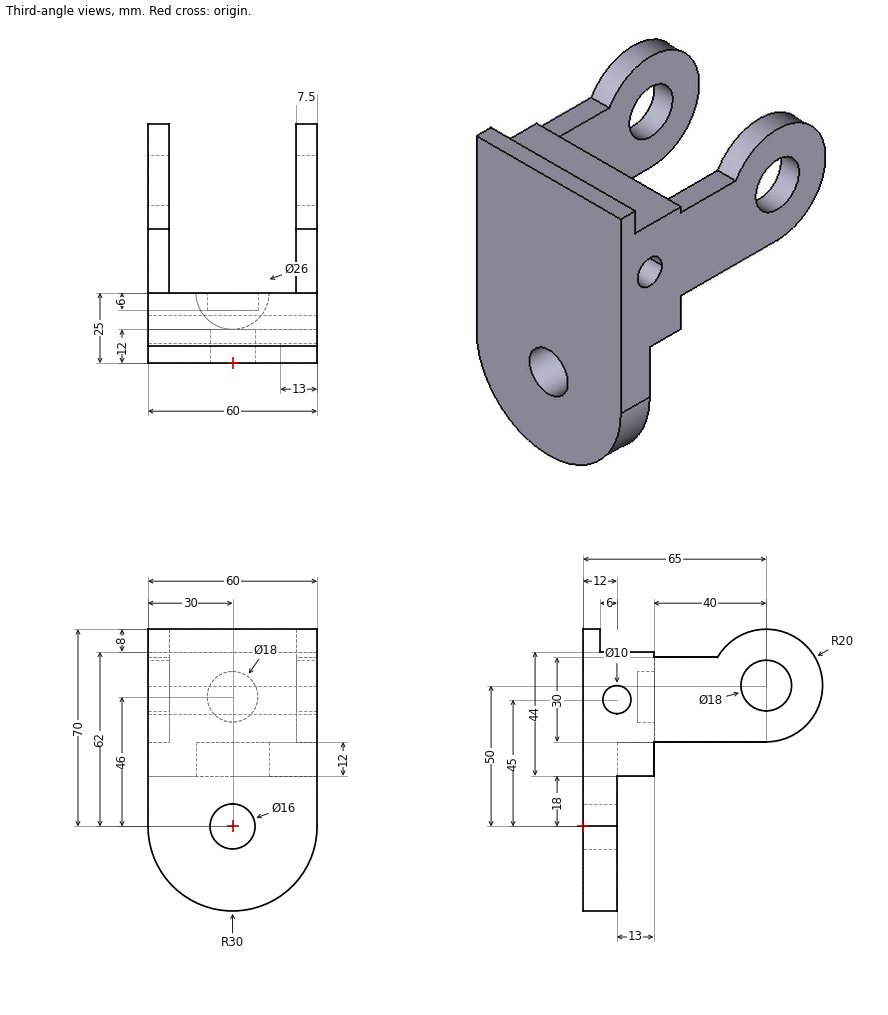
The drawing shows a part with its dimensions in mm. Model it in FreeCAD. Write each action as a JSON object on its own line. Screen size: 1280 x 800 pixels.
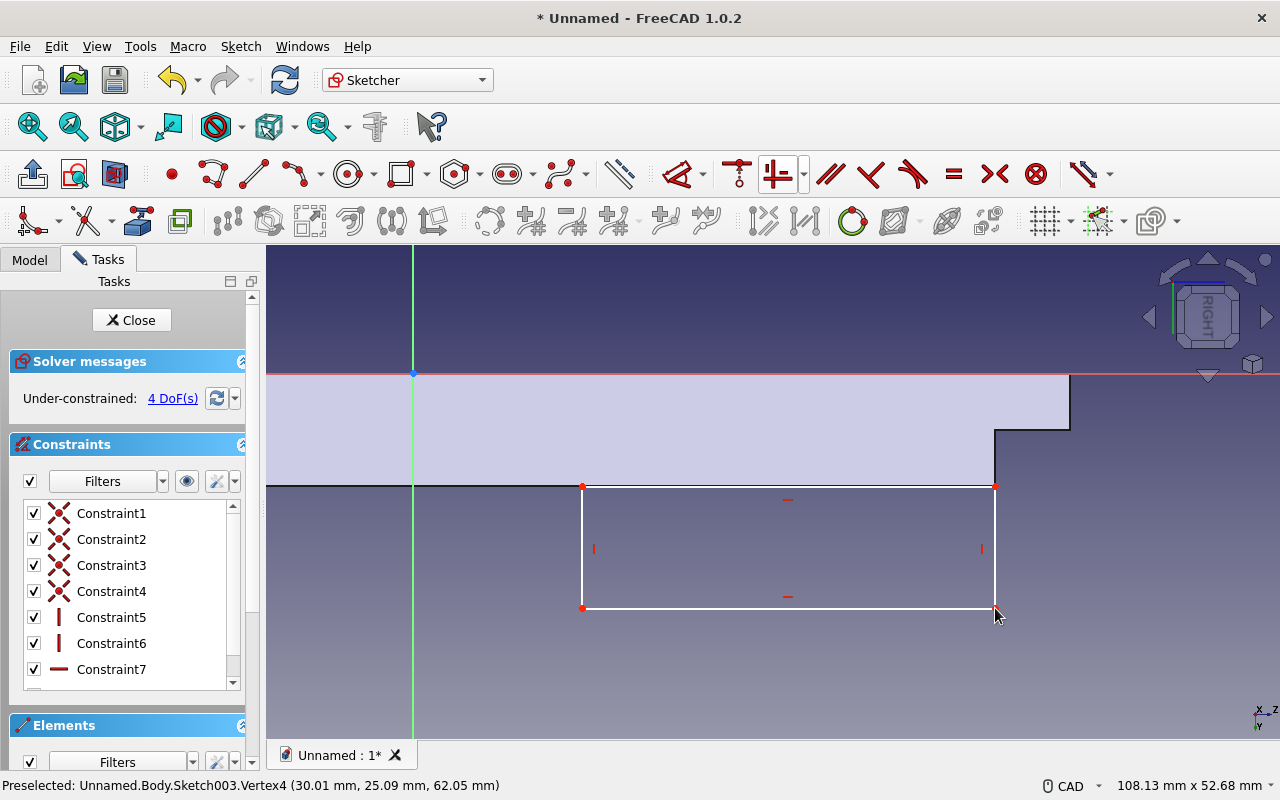
{"action": "key", "text": "d"}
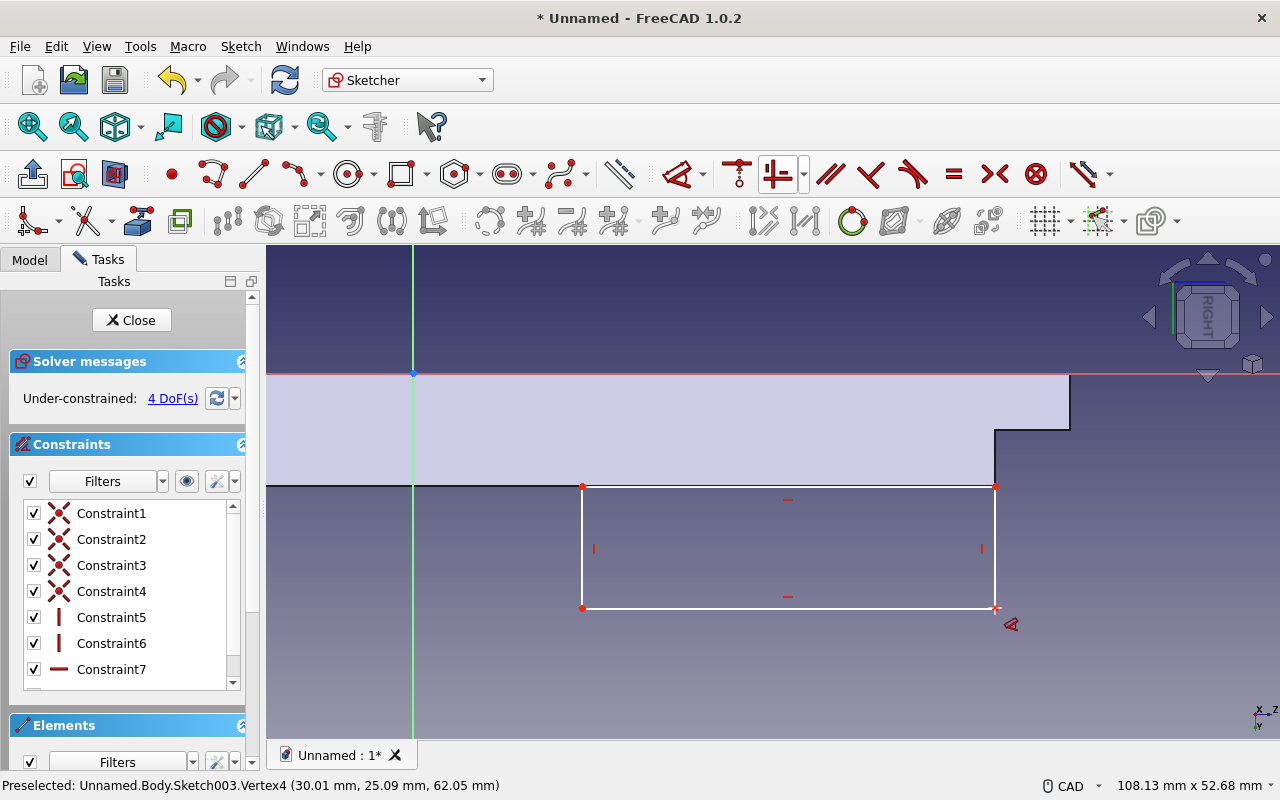
{"action": "left_click", "coordinate": [582, 524]}
{"action": "left_click", "coordinate": [548, 548]}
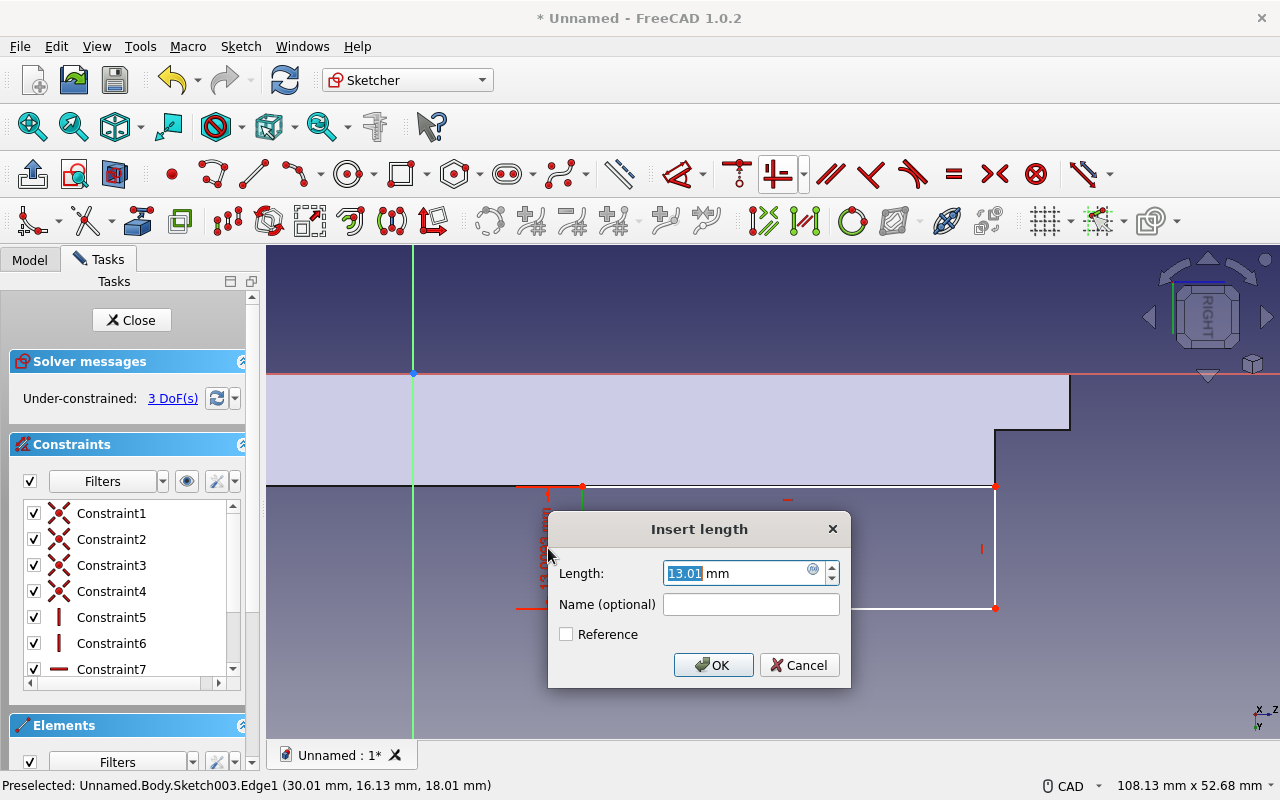
{"action": "type", "text": "13"}
{"action": "key", "text": "Return"}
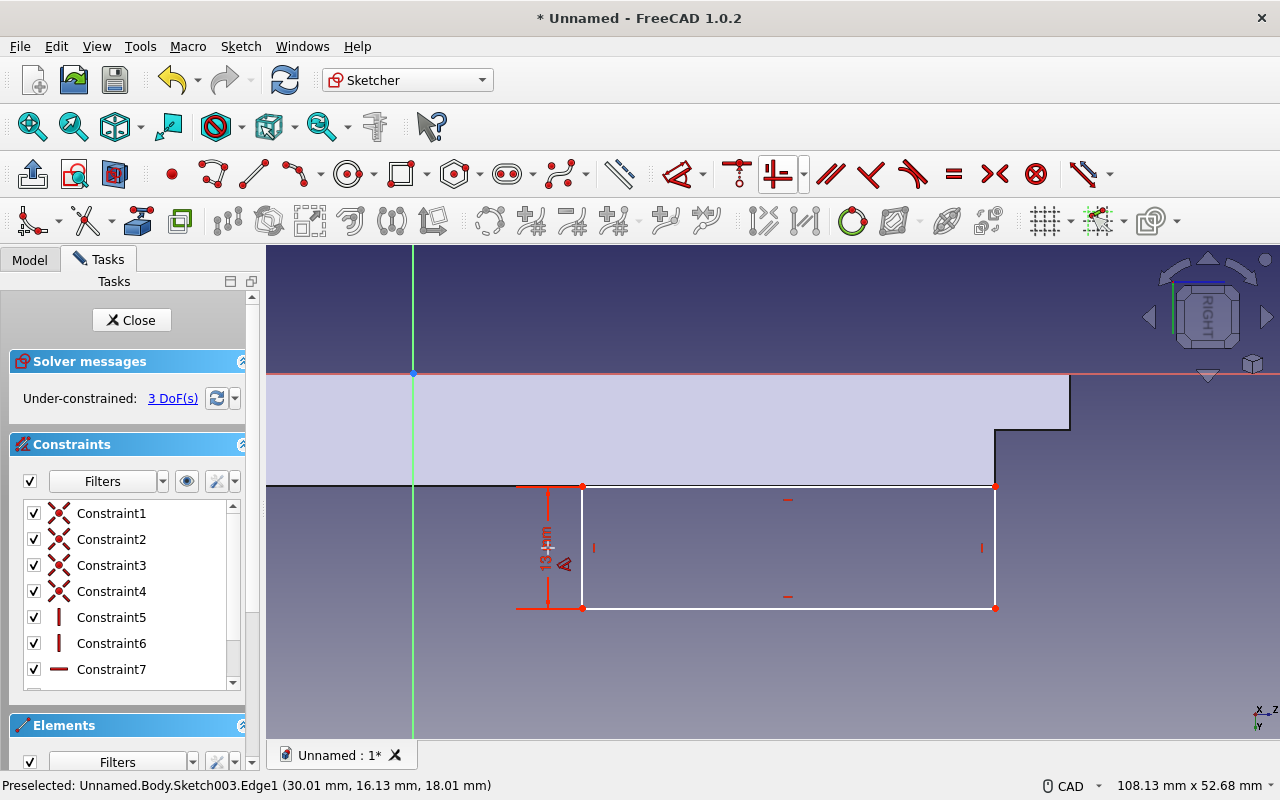
{"action": "left_click", "coordinate": [706, 609]}
{"action": "left_click", "coordinate": [788, 643]}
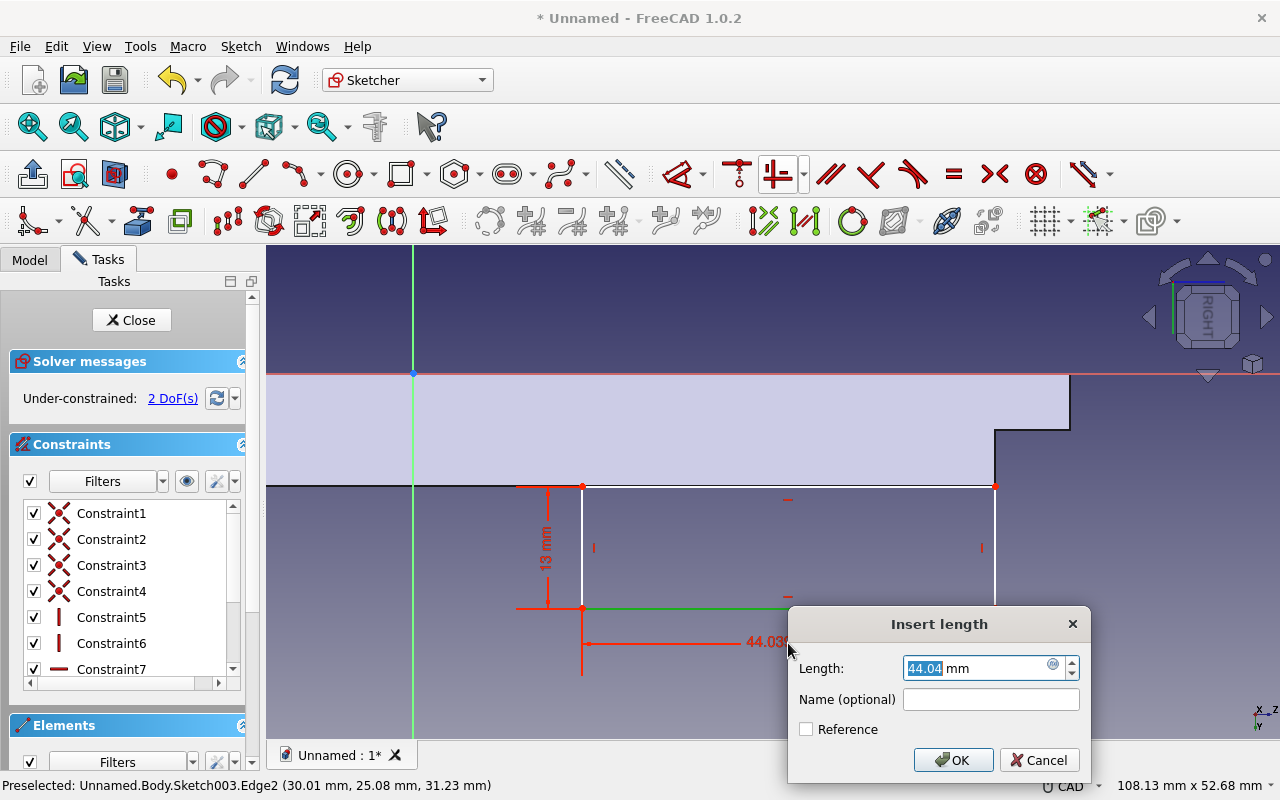
{"action": "type", "text": "44"}
{"action": "key", "text": "Return"}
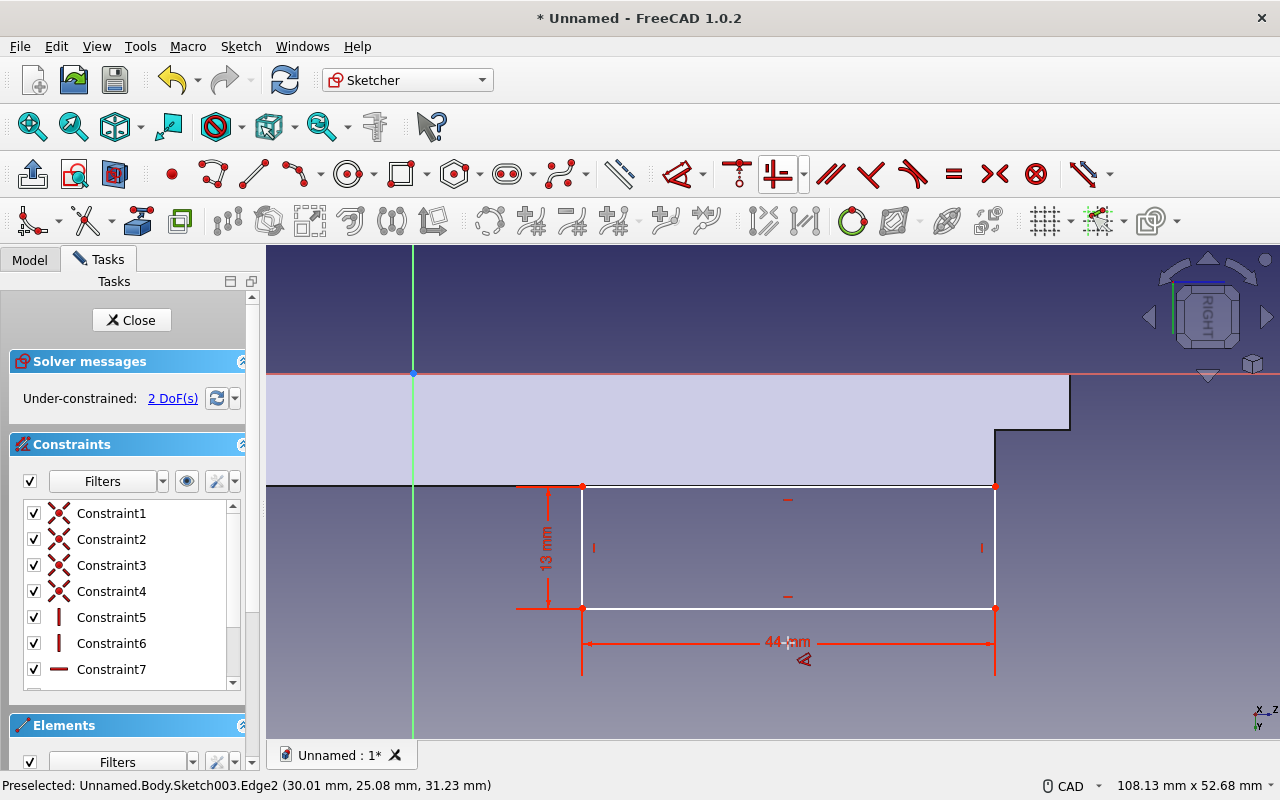
{"action": "left_click", "coordinate": [582, 487]}
{"action": "left_click", "coordinate": [498, 340]}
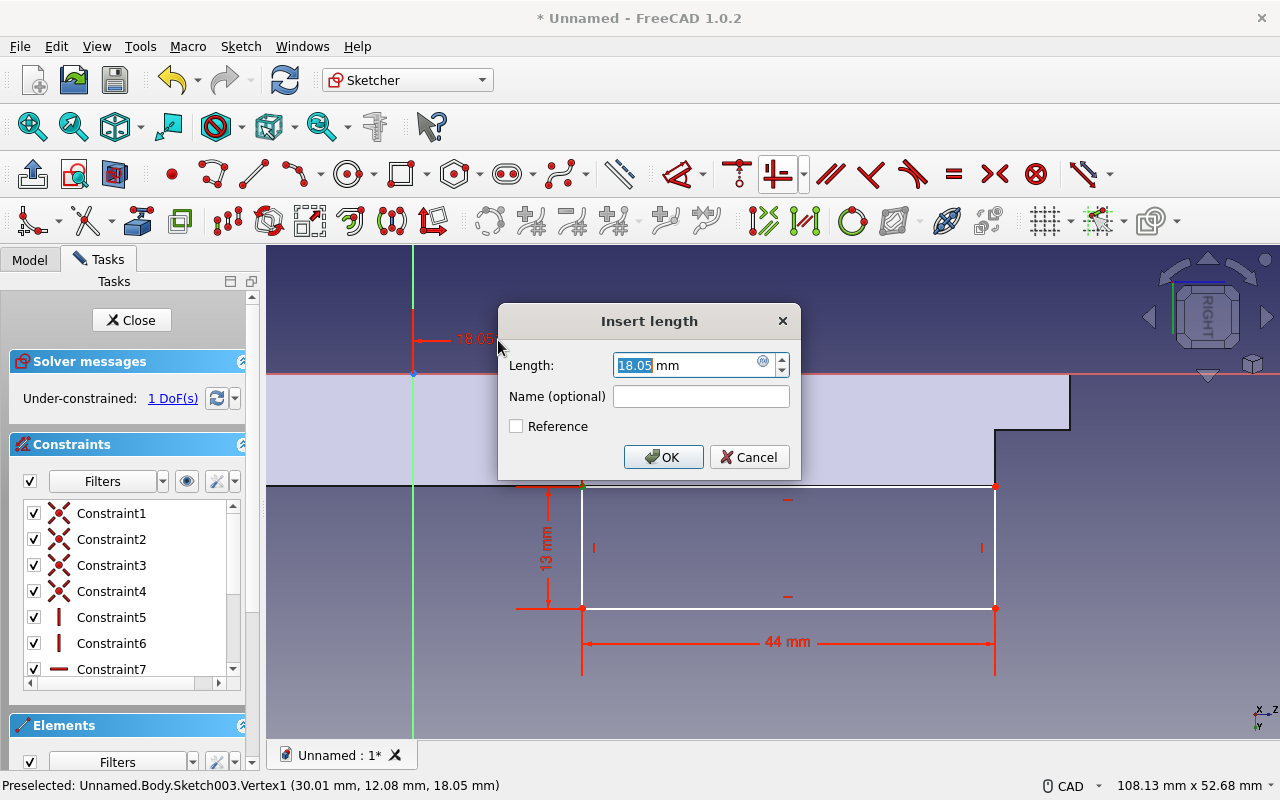
{"action": "type", "text": "18"}
{"action": "key", "text": "Return"}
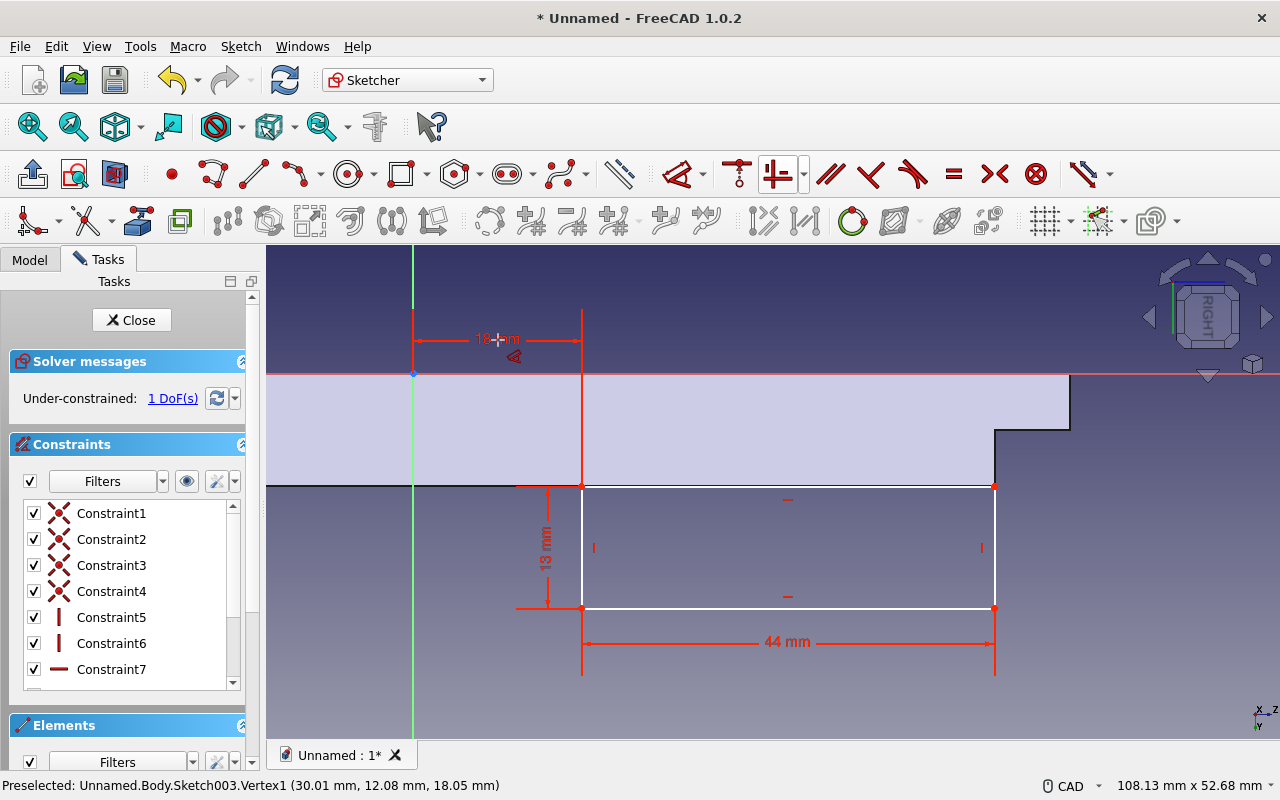
{"action": "left_click", "coordinate": [582, 487]}
{"action": "left_click", "coordinate": [379, 430]}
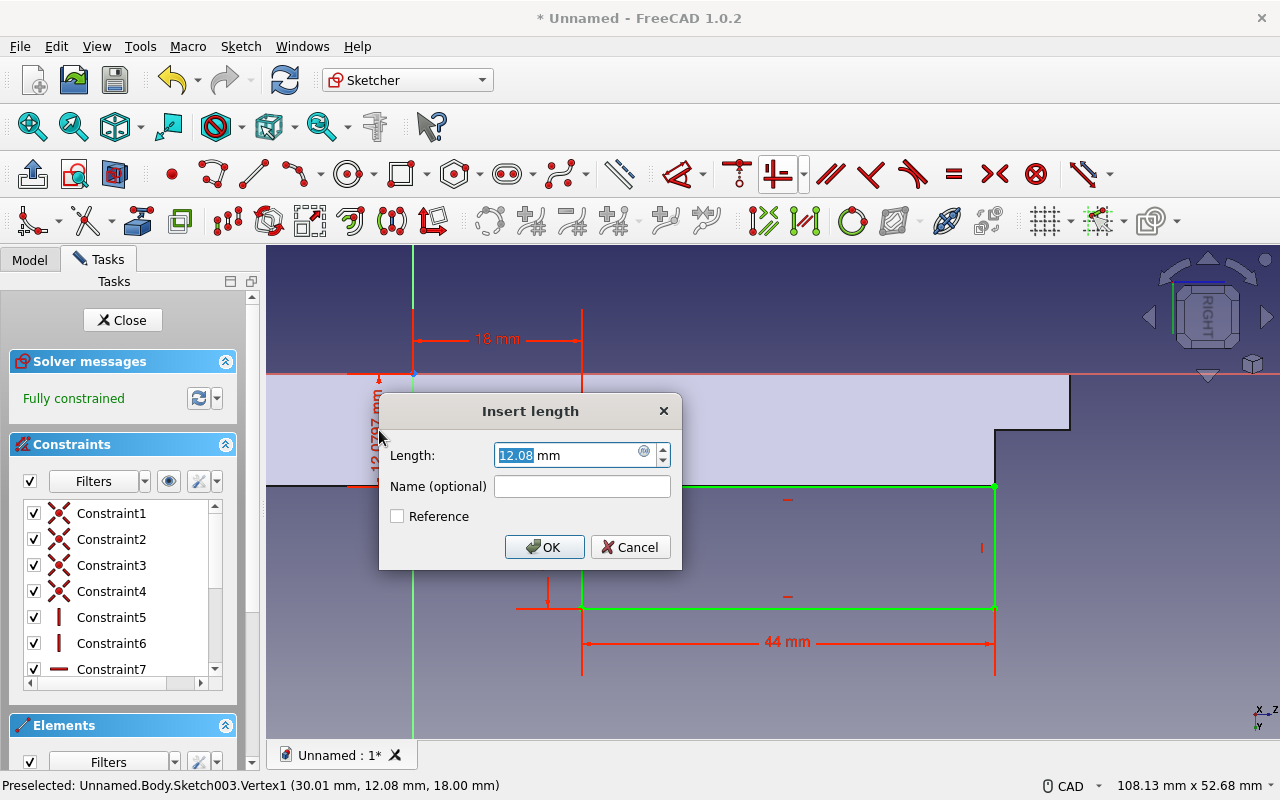
{"action": "type", "text": "12"}
{"action": "key", "text": "Return"}
{"action": "key", "text": "Escape"}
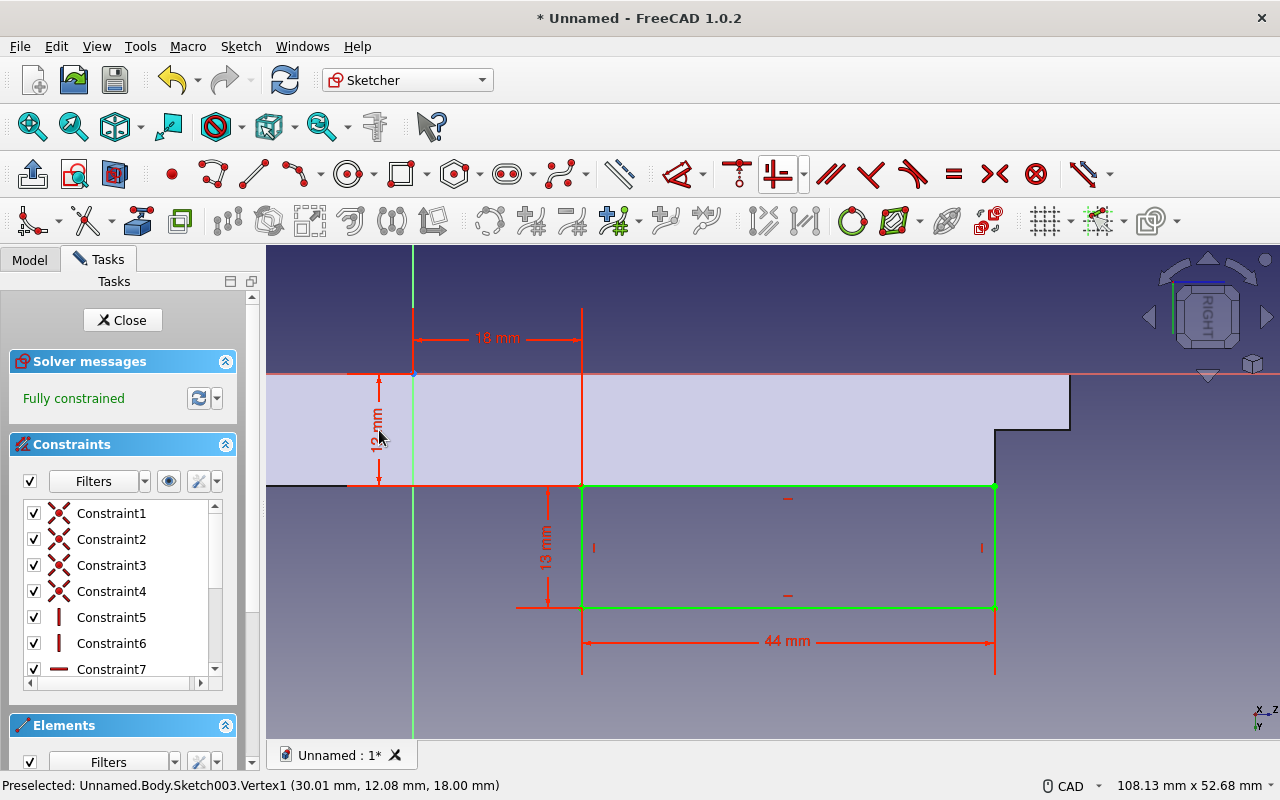
{"action": "left_click", "coordinate": [123, 320]}